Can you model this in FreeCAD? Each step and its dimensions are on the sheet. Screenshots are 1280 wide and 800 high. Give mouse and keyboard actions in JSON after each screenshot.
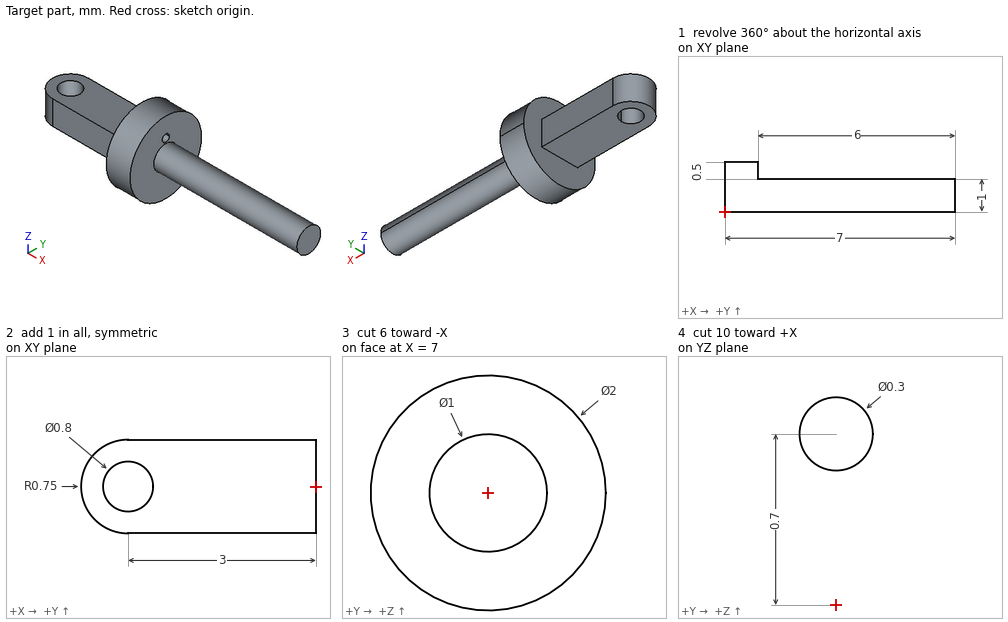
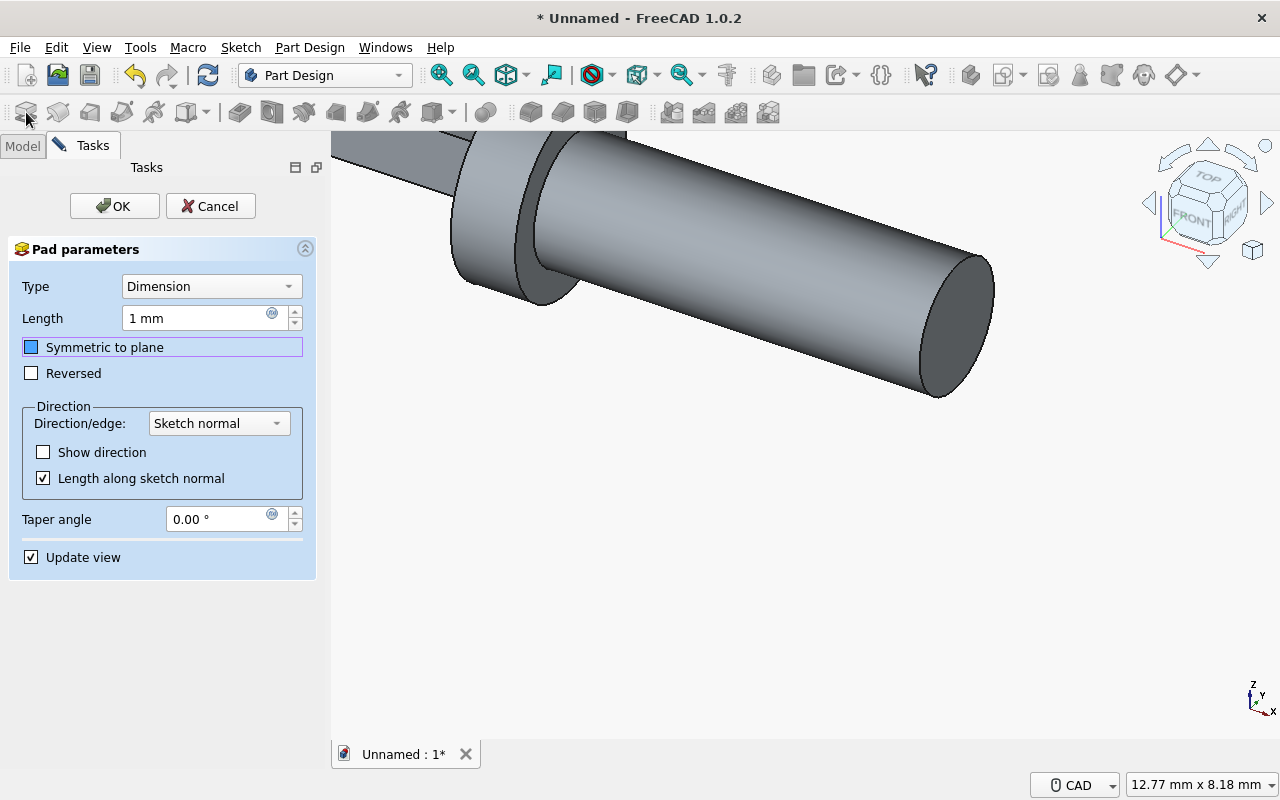
{"action": "left_click", "coordinate": [30, 347]}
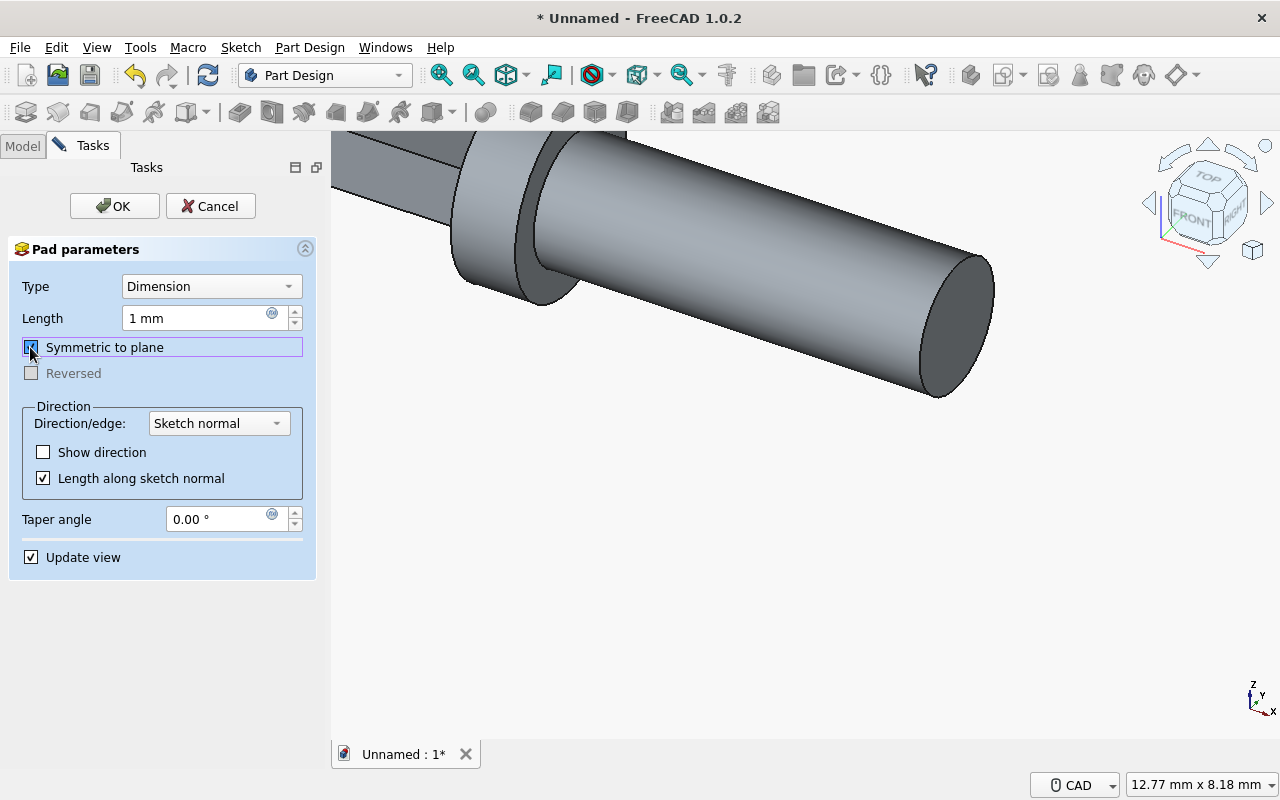
{"action": "left_click", "coordinate": [115, 206]}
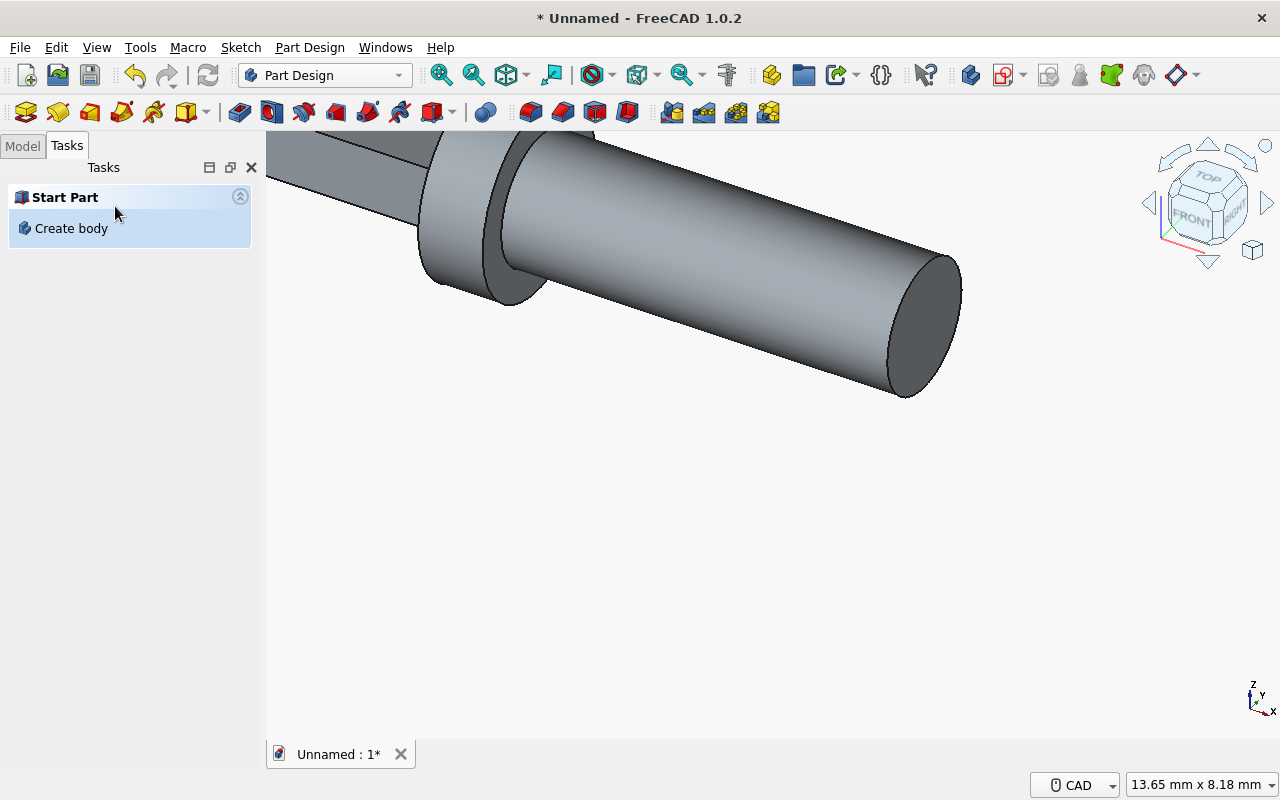
{"action": "left_click", "coordinate": [442, 76]}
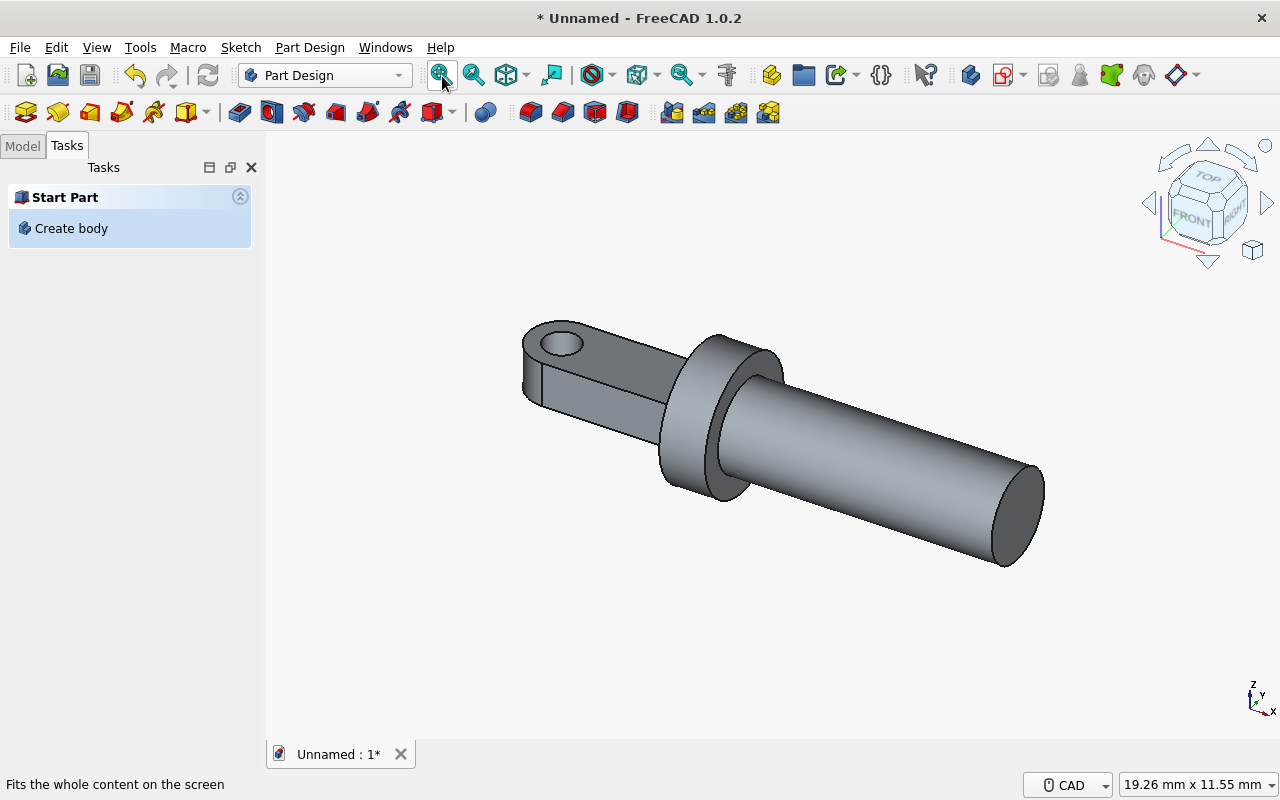
{"action": "left_click", "coordinate": [1018, 515]}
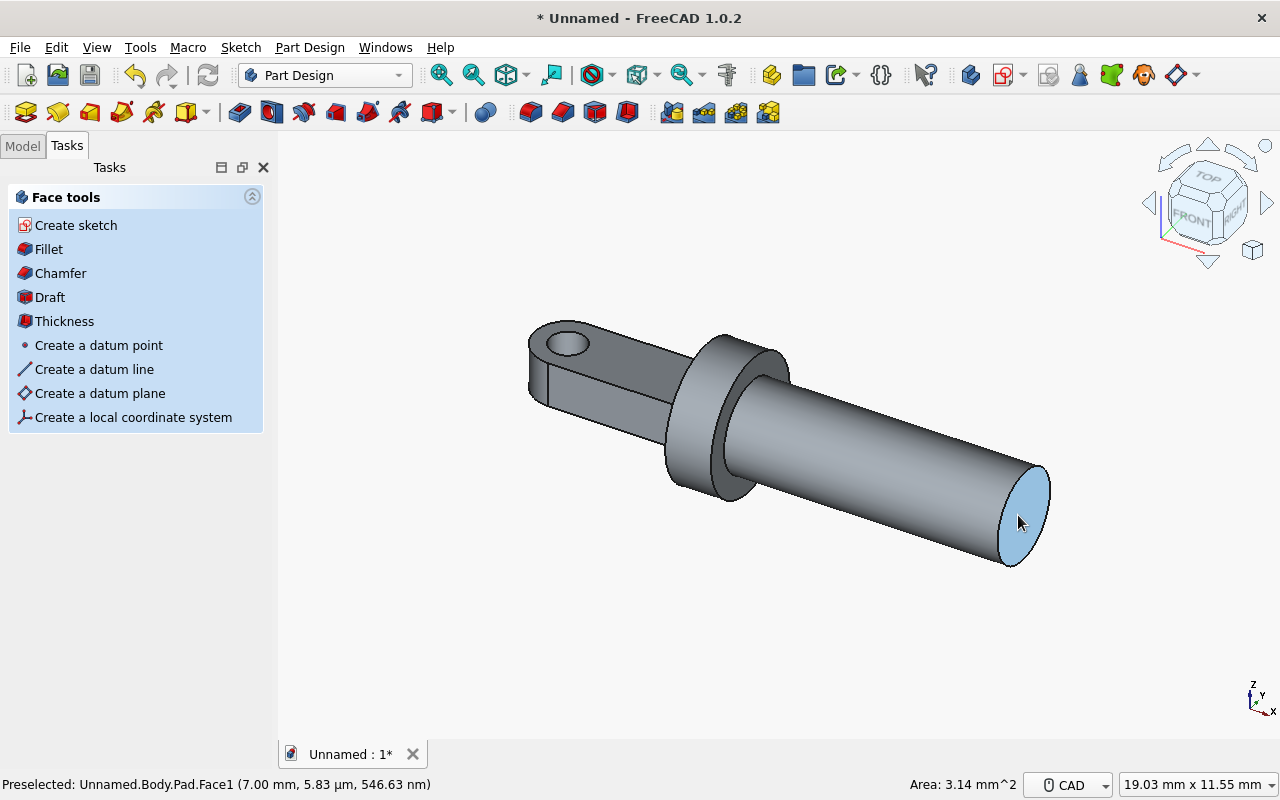
{"action": "left_click", "coordinate": [1004, 76]}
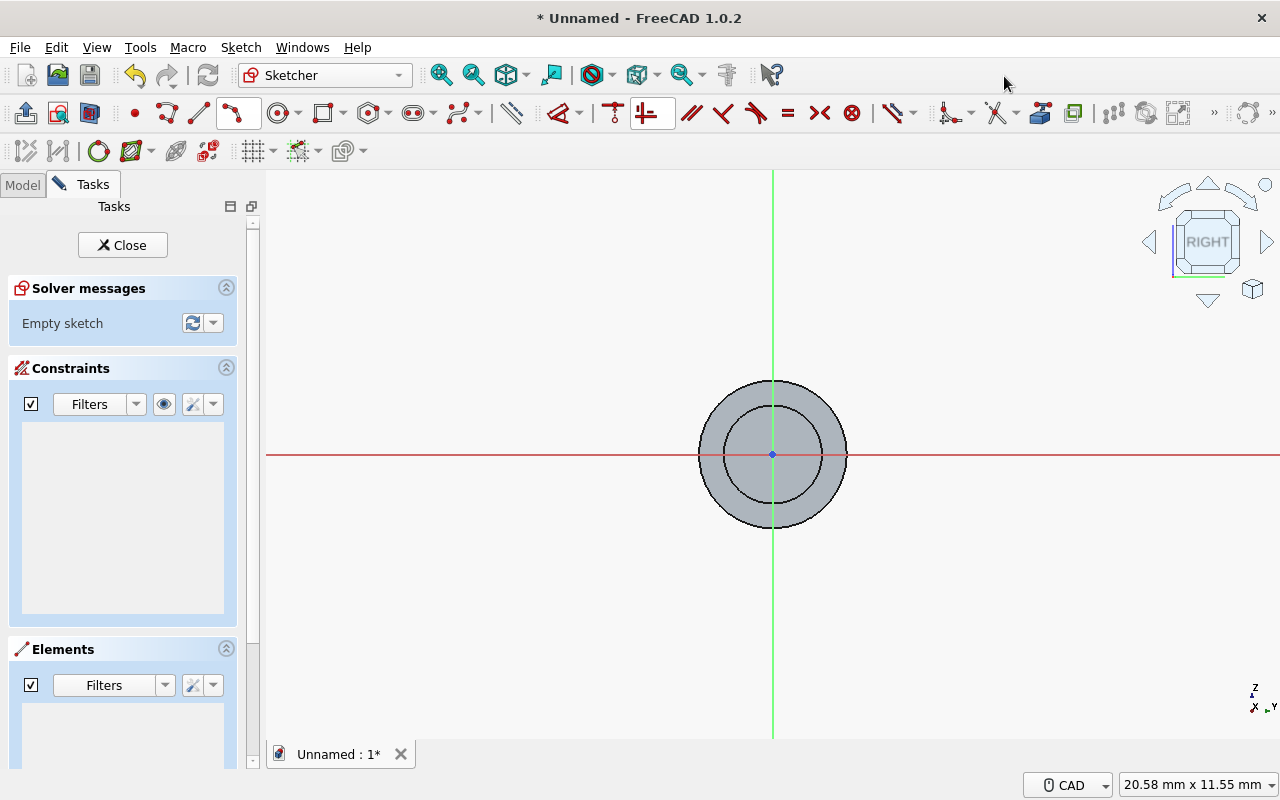
{"action": "scroll", "coordinate": [795, 454], "scroll_direction": "up", "scroll_amount": 7}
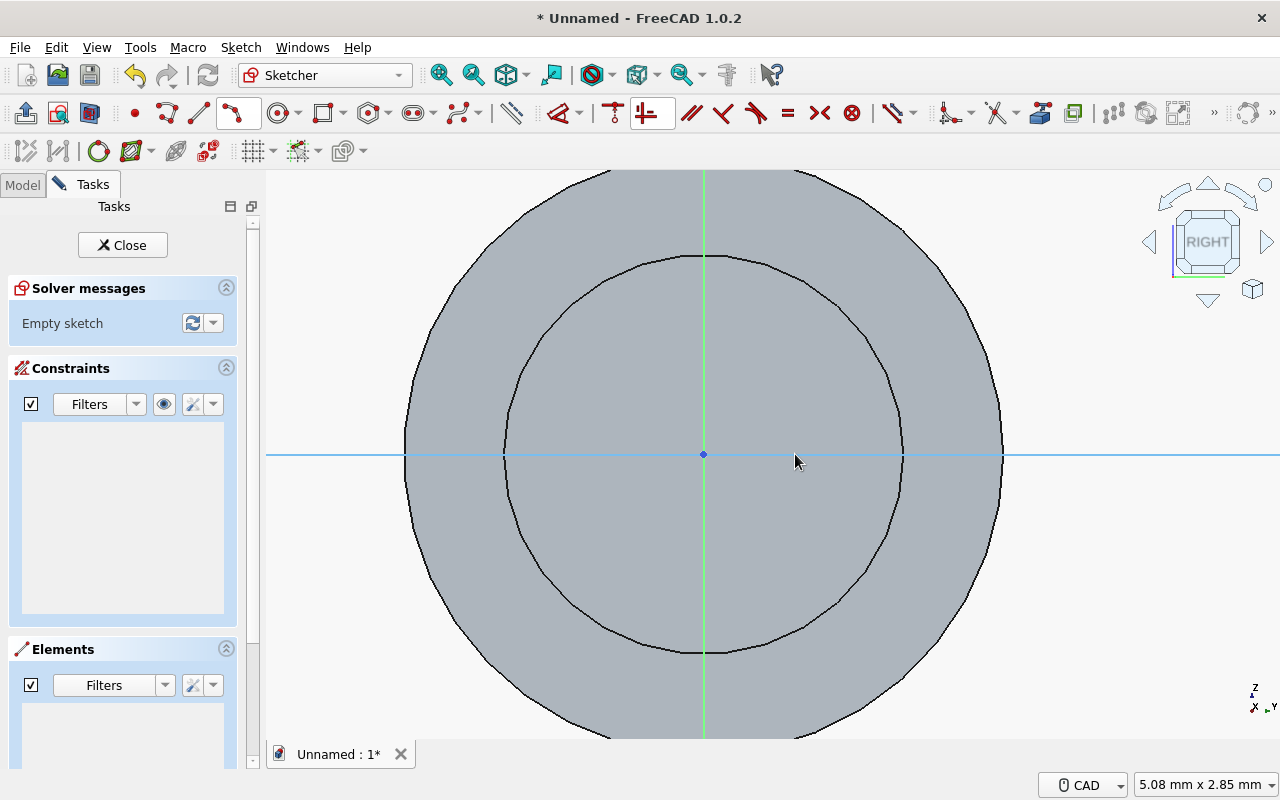
{"action": "left_click", "coordinate": [278, 114]}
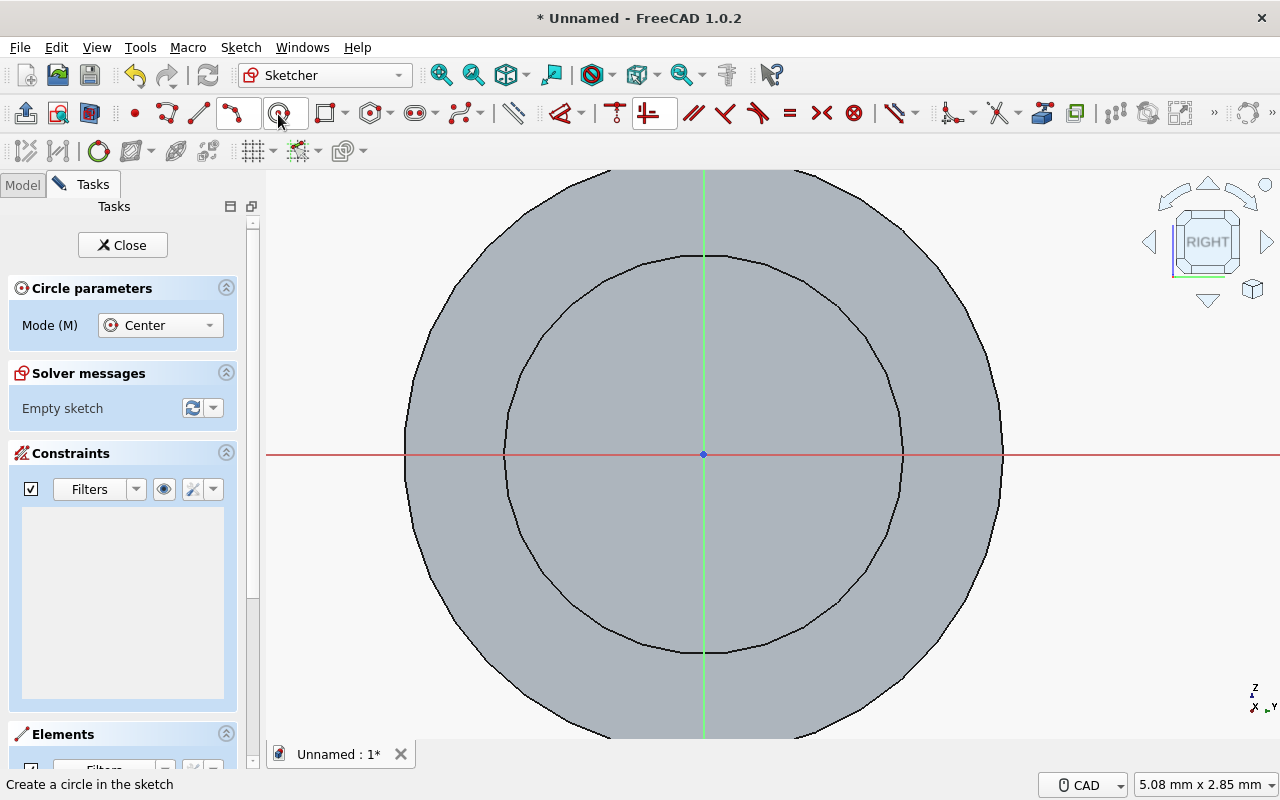
{"action": "left_click", "coordinate": [704, 454]}
{"action": "left_click", "coordinate": [845, 313]}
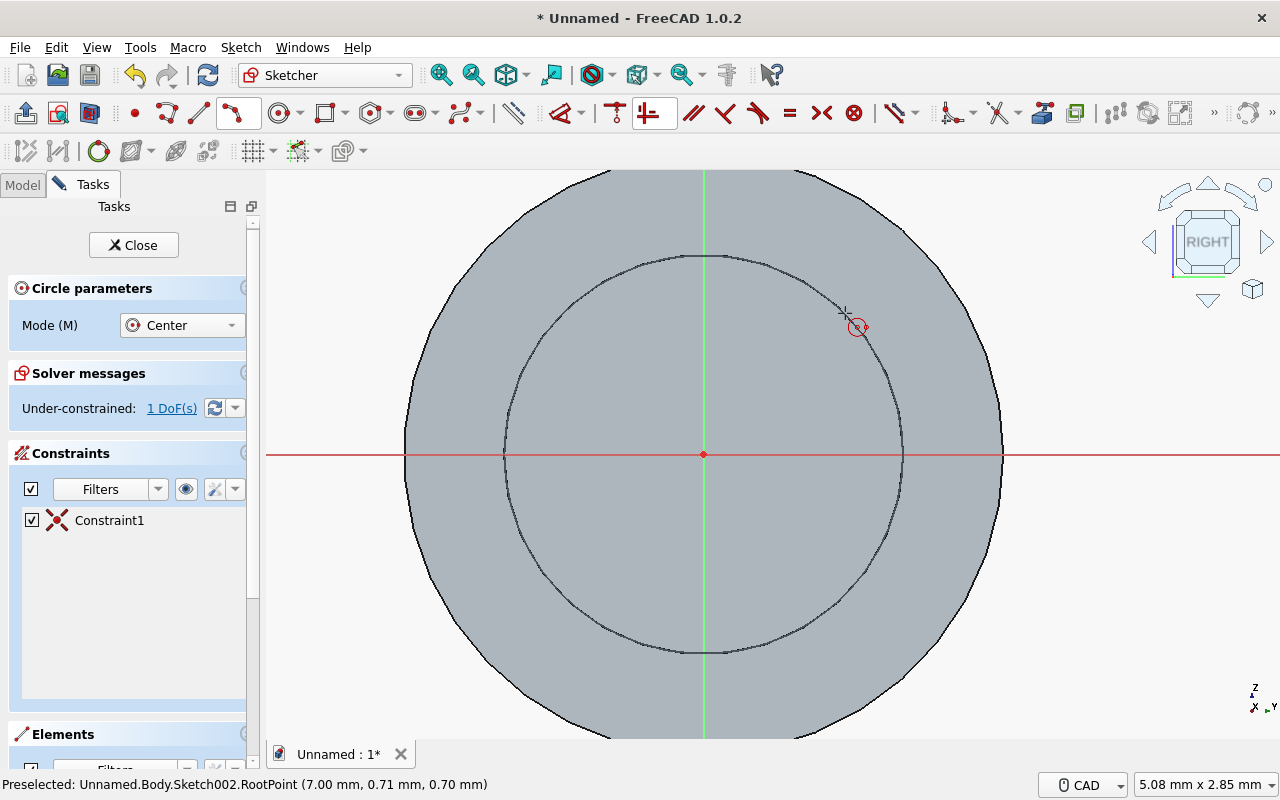
{"action": "left_click", "coordinate": [704, 454]}
{"action": "left_click", "coordinate": [774, 384]}
{"action": "key", "text": "Escape"}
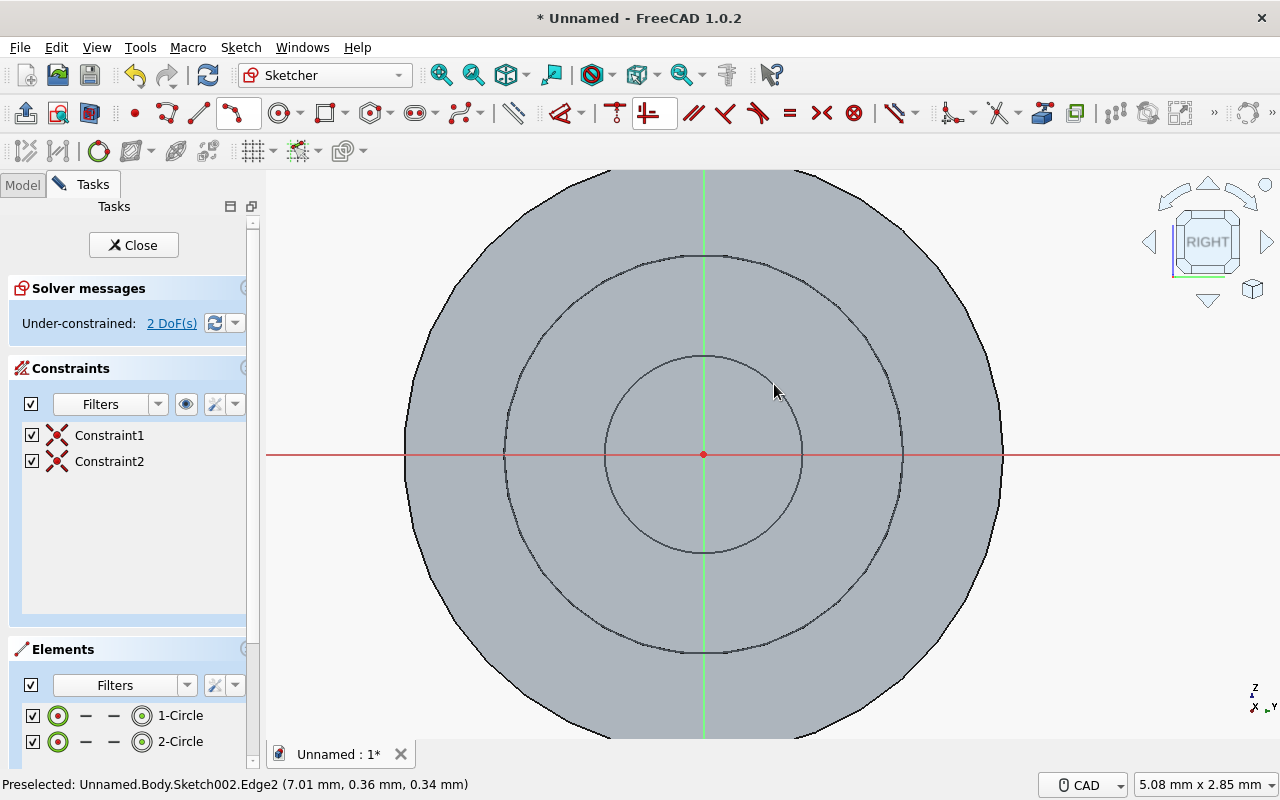
{"action": "left_click", "coordinate": [560, 114]}